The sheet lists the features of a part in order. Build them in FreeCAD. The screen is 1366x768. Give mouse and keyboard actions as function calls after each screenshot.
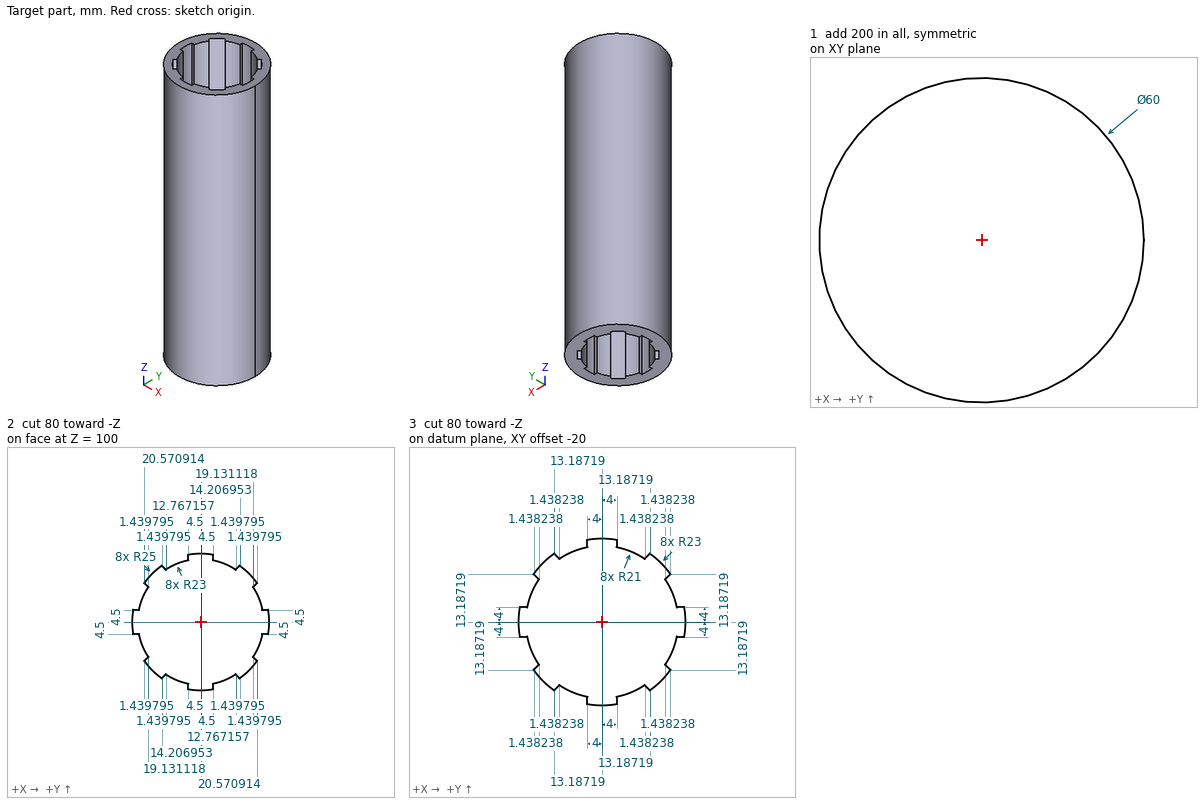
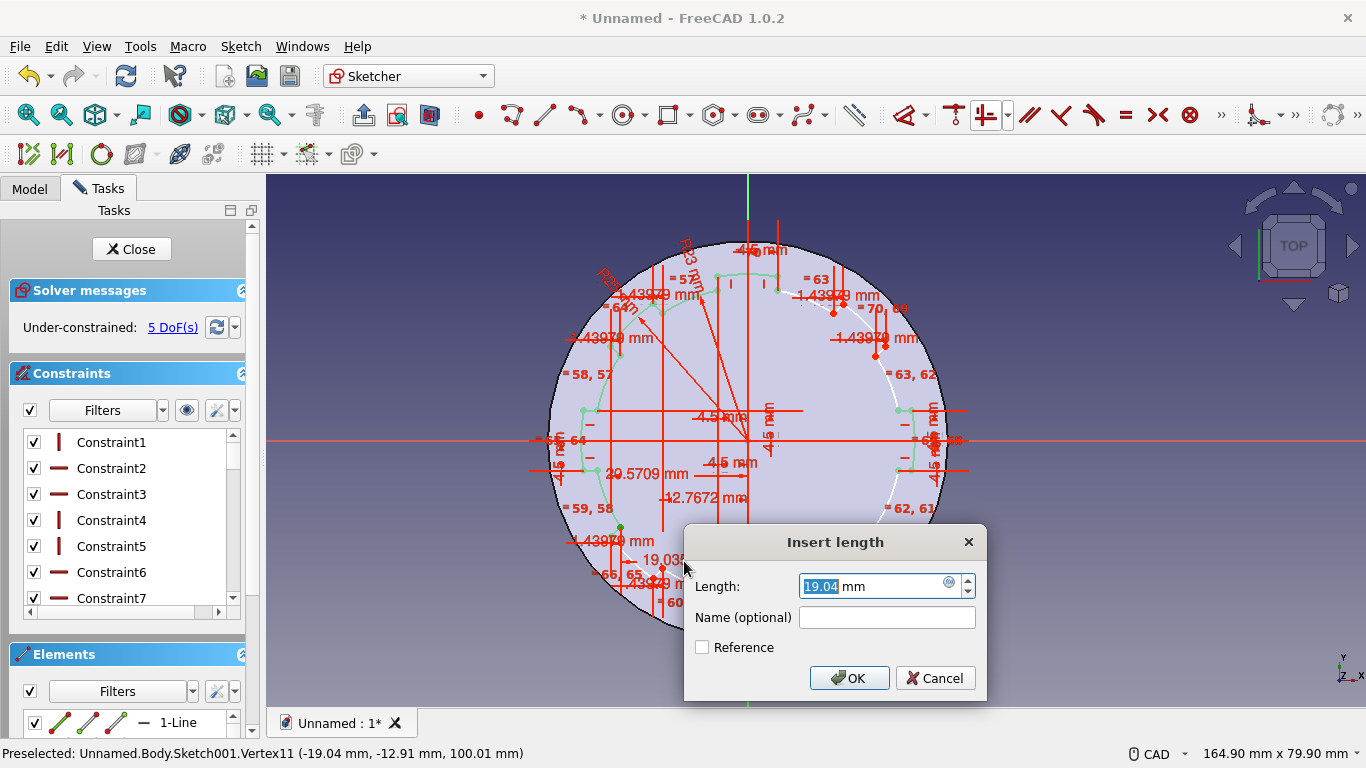
text(19.131118)
key(Return)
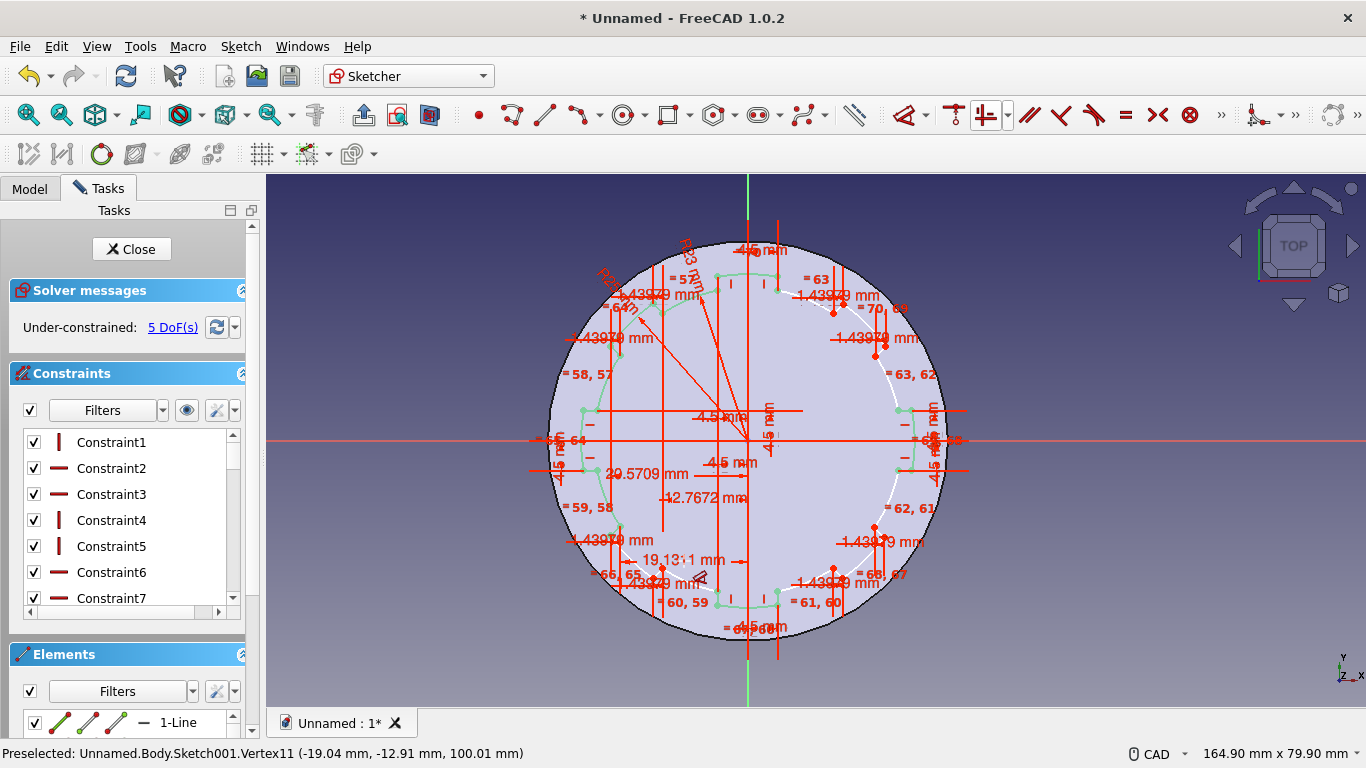
click(653, 578)
click(679, 612)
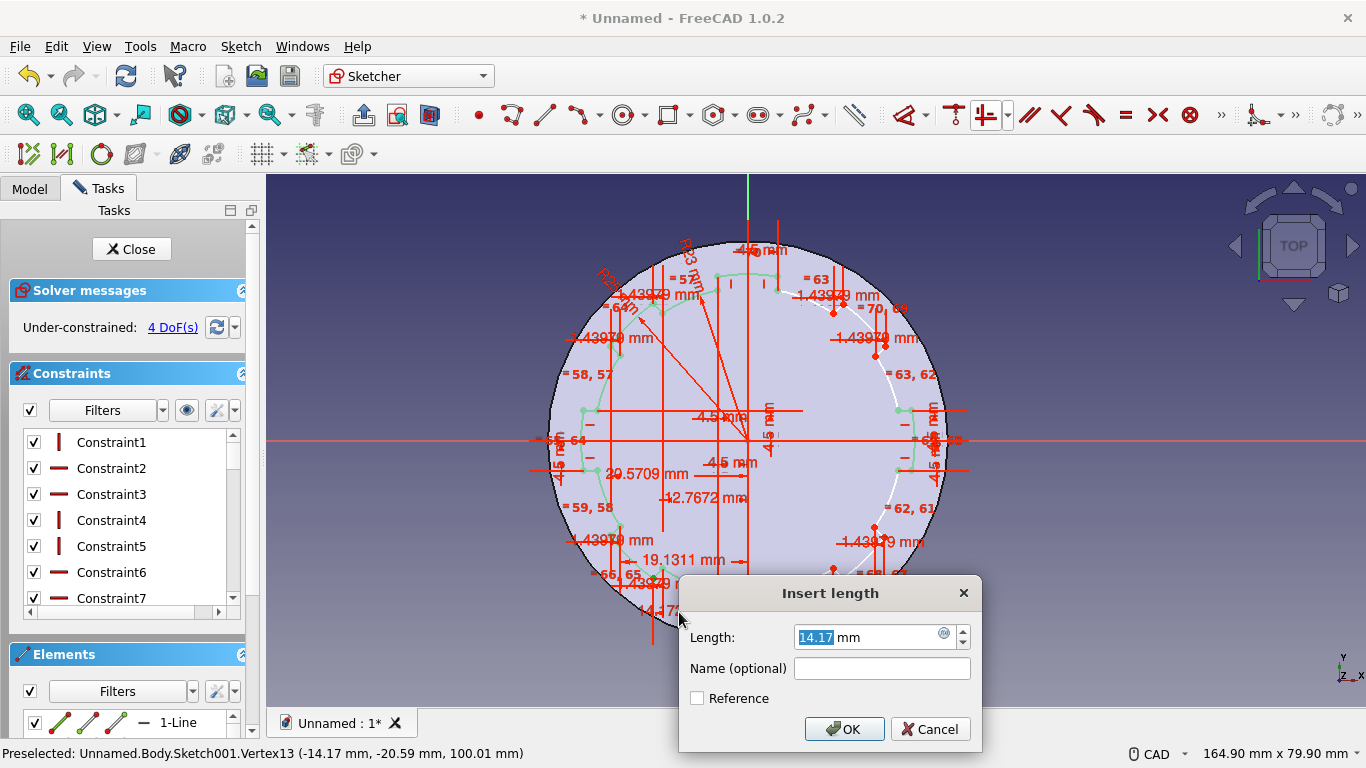
text(14.206953)
key(Return)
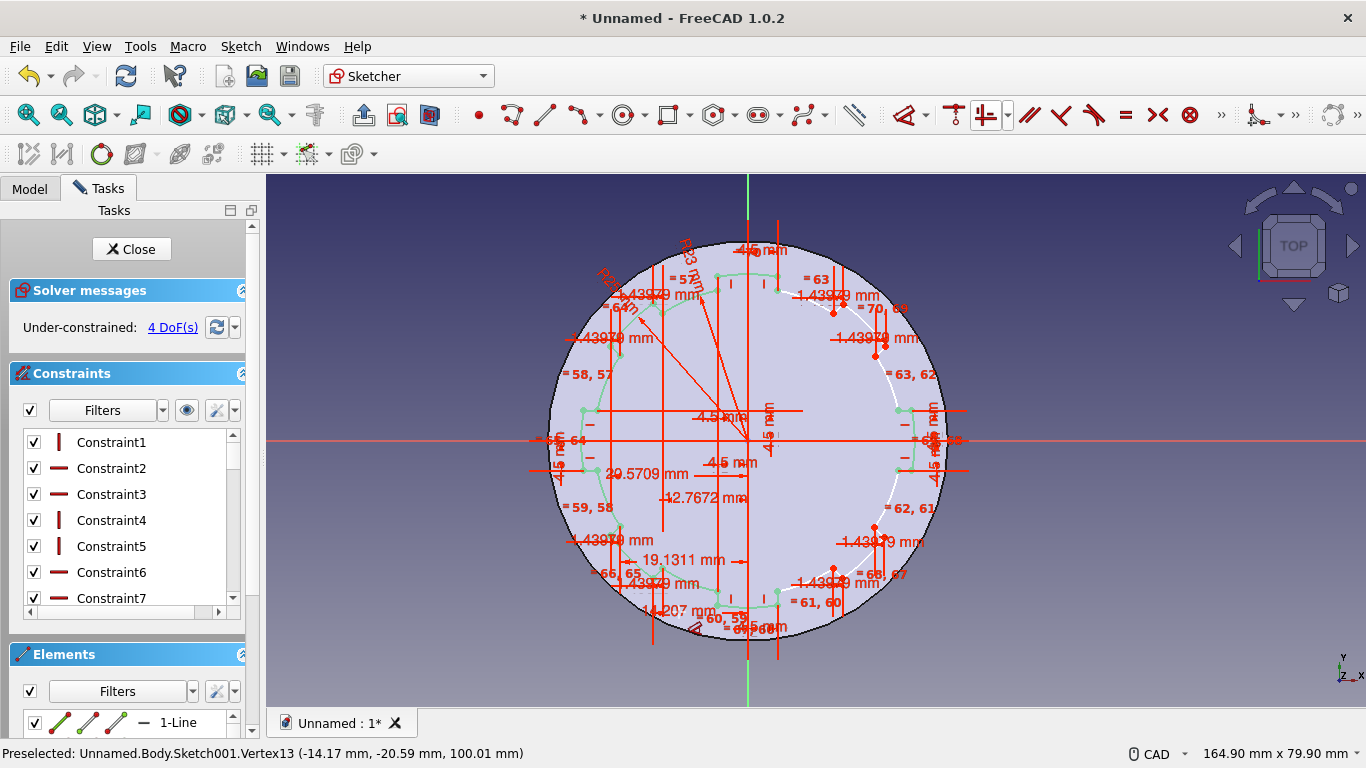
click(833, 569)
click(791, 383)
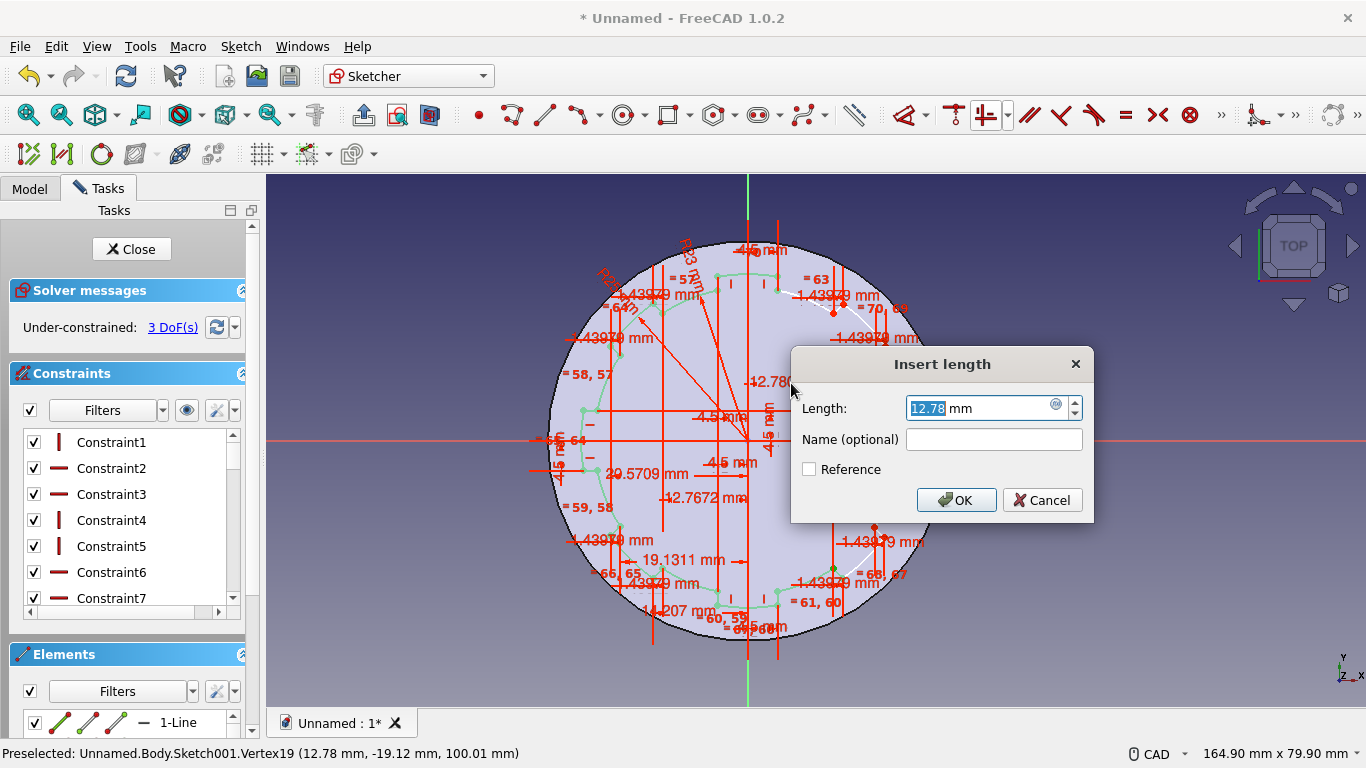
text(12.767157)
key(Return)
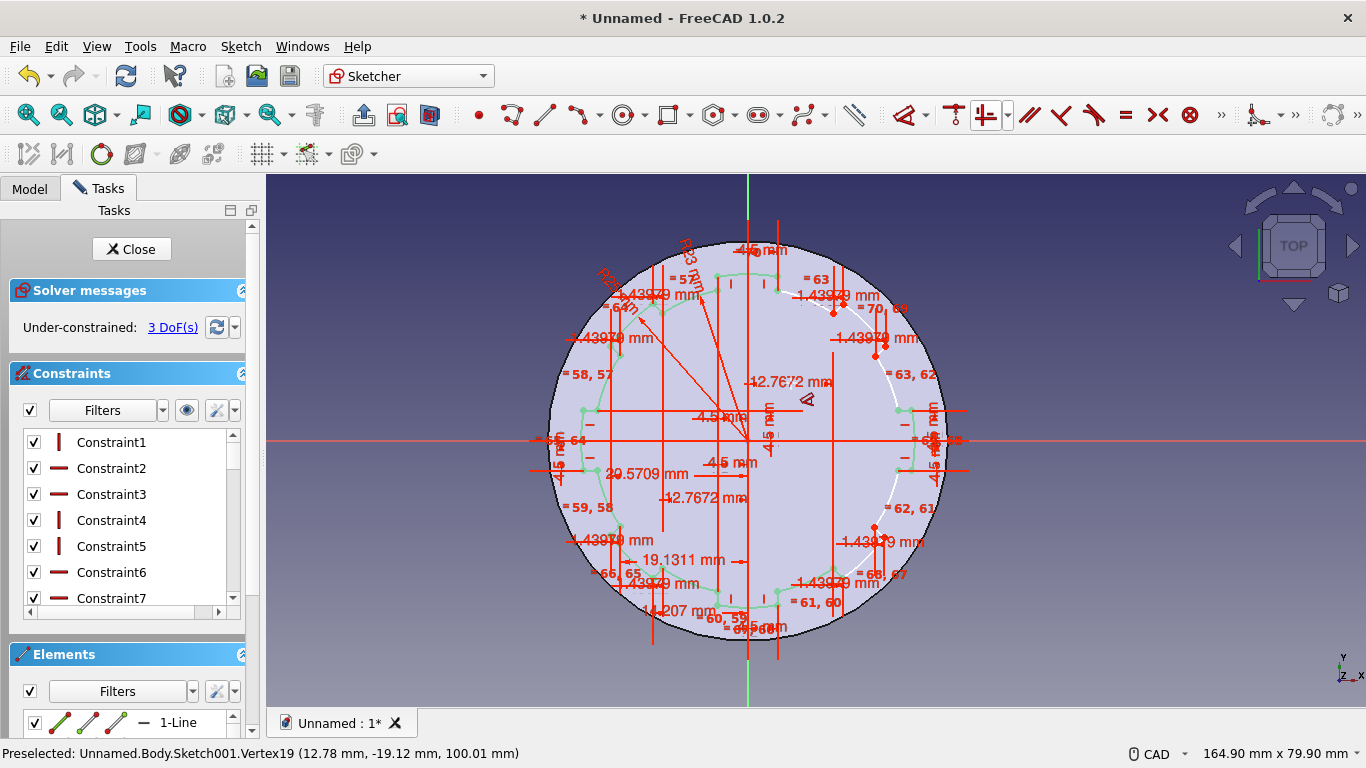
click(884, 537)
click(847, 407)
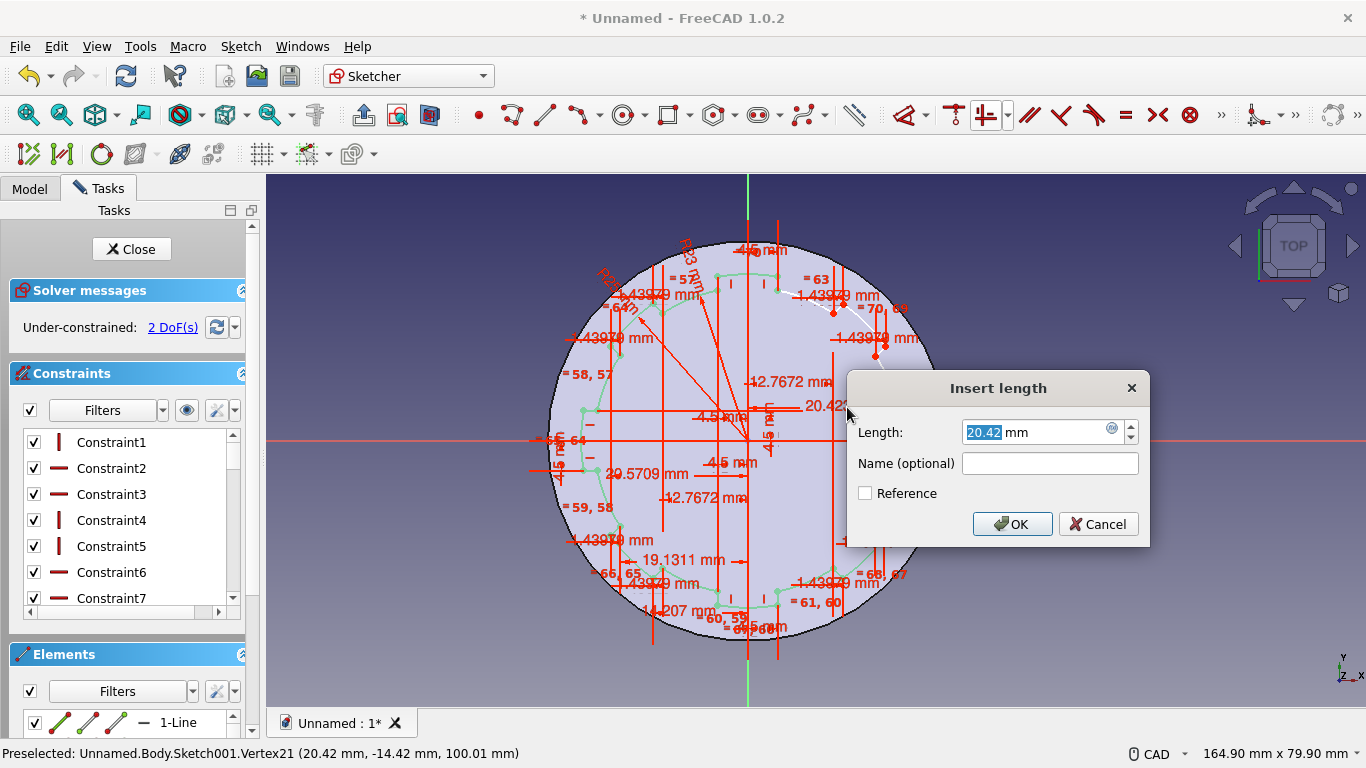
text(20.570914)
key(Return)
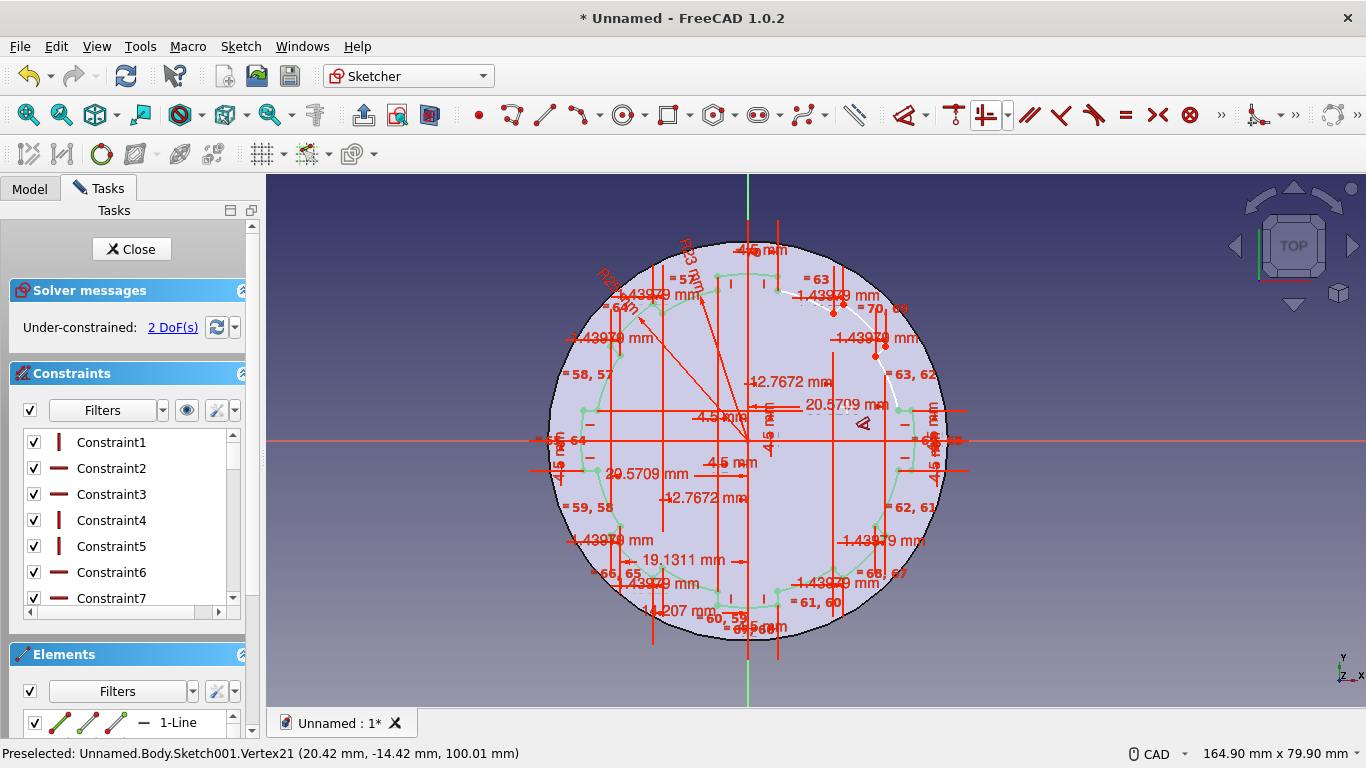
click(876, 356)
click(782, 322)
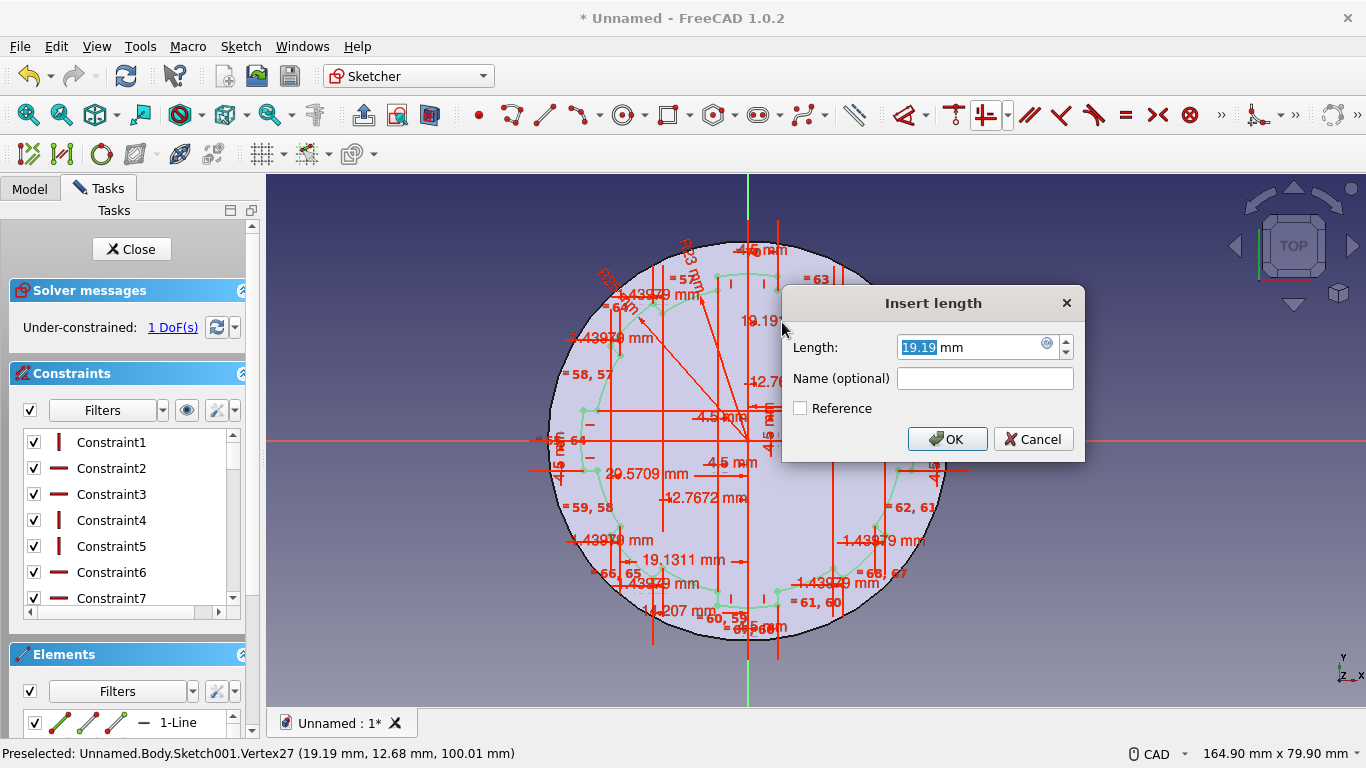
text(19.131118)
key(Return)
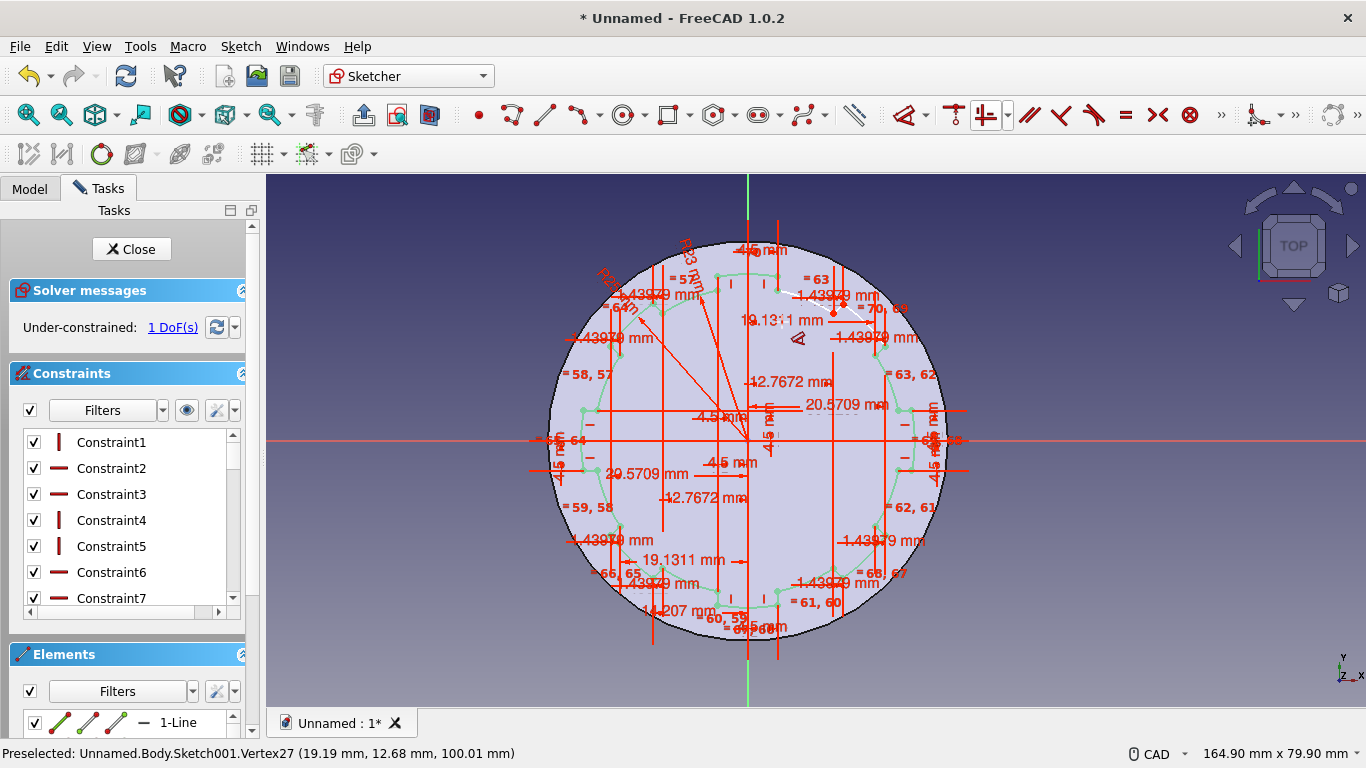
click(843, 304)
click(817, 475)